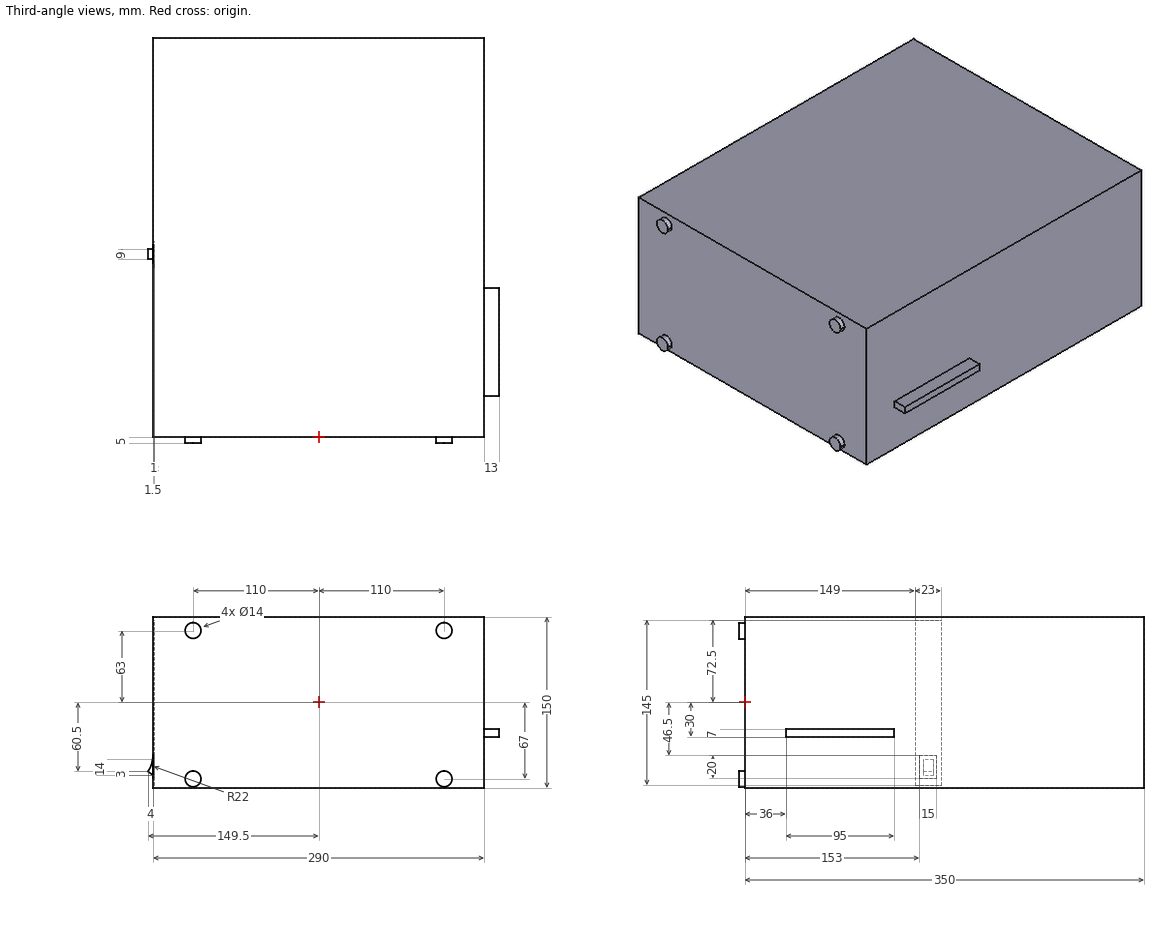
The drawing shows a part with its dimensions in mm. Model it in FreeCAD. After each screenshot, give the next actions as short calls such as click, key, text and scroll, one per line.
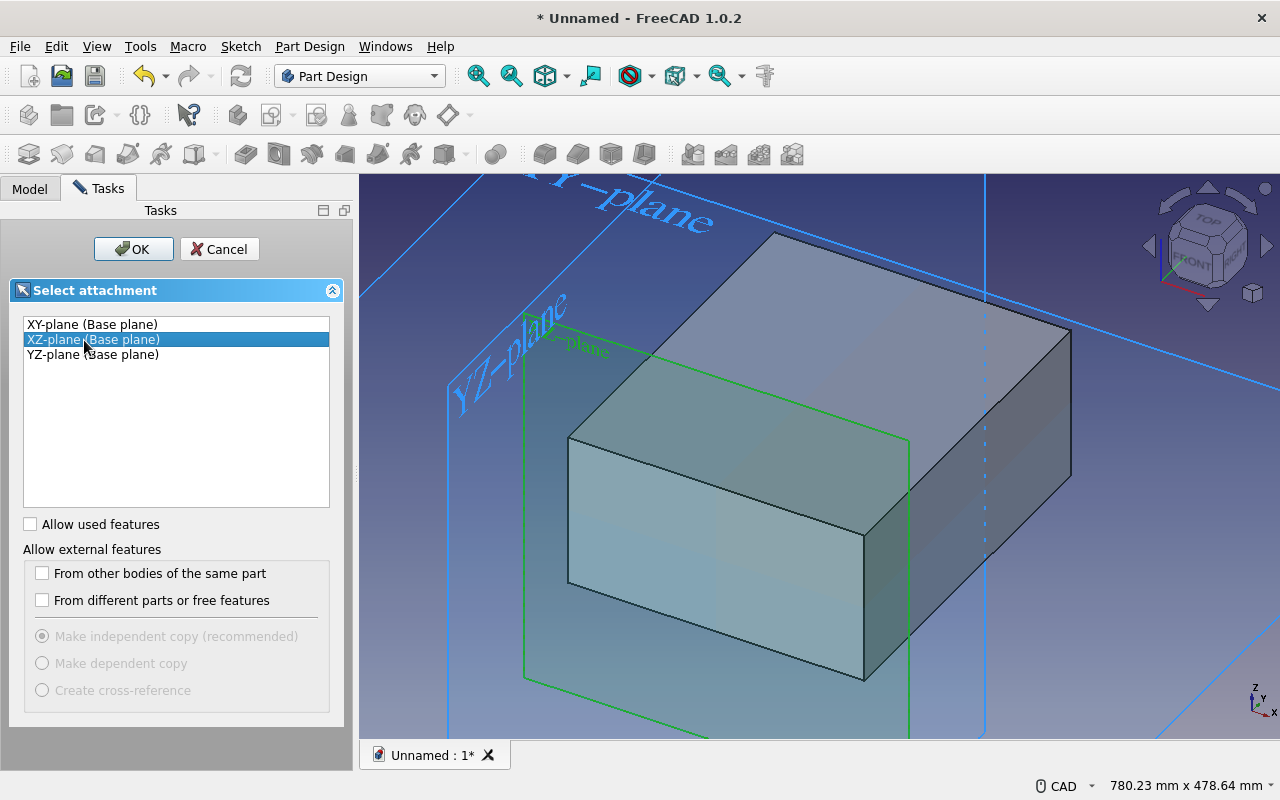
click(134, 249)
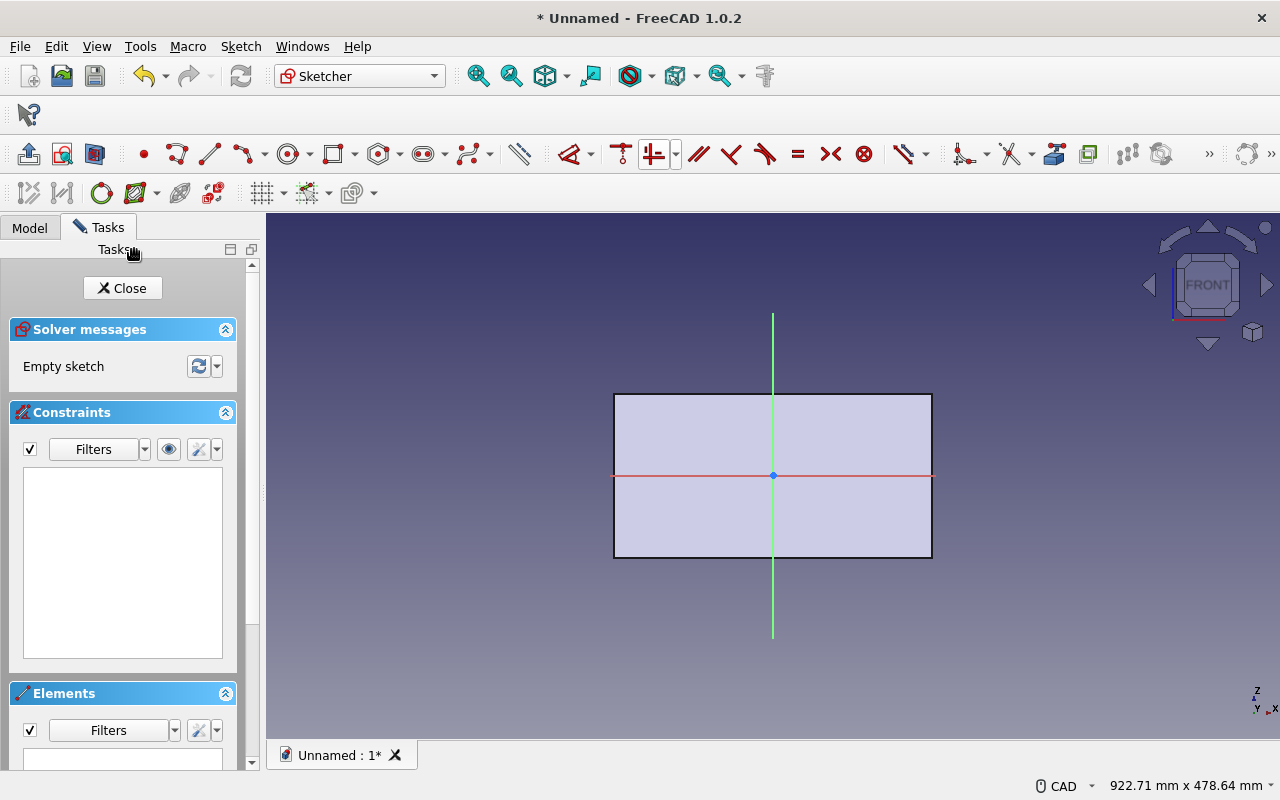
scroll(829, 480, up, 4)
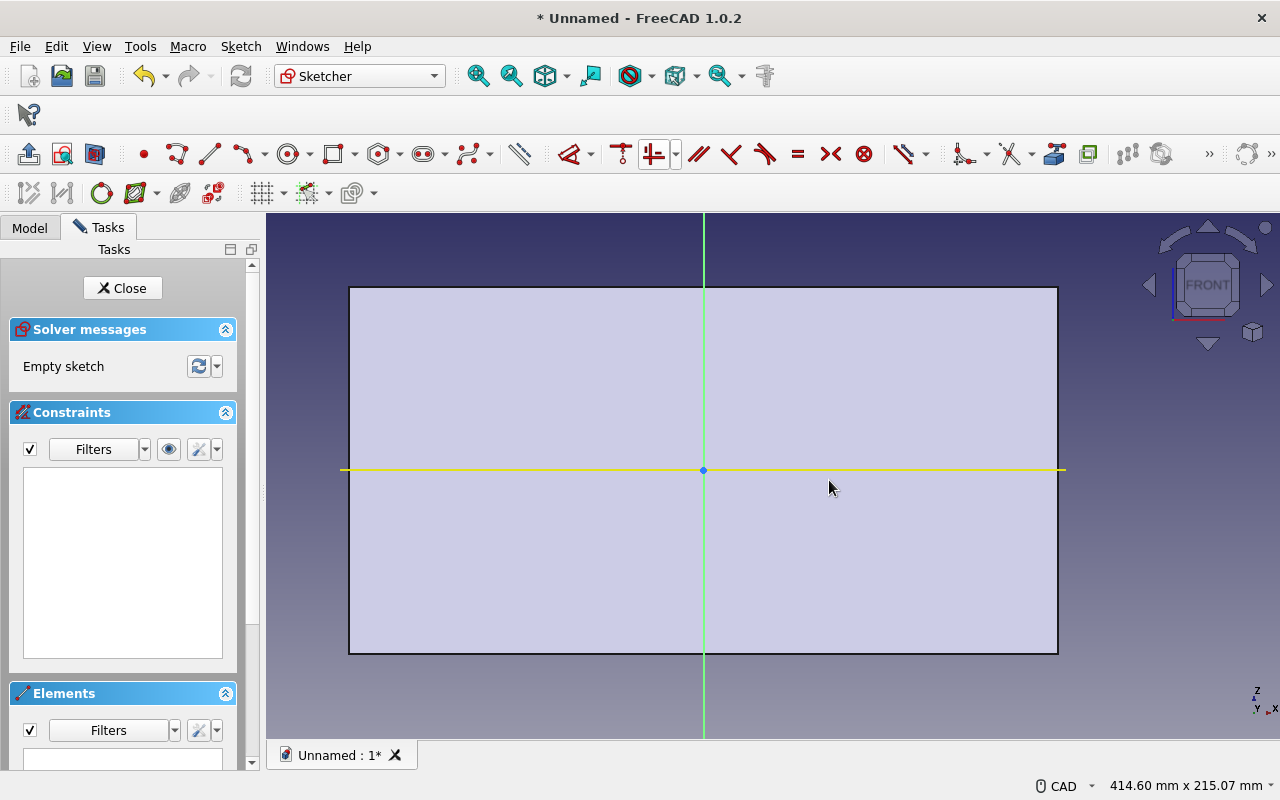
click(288, 154)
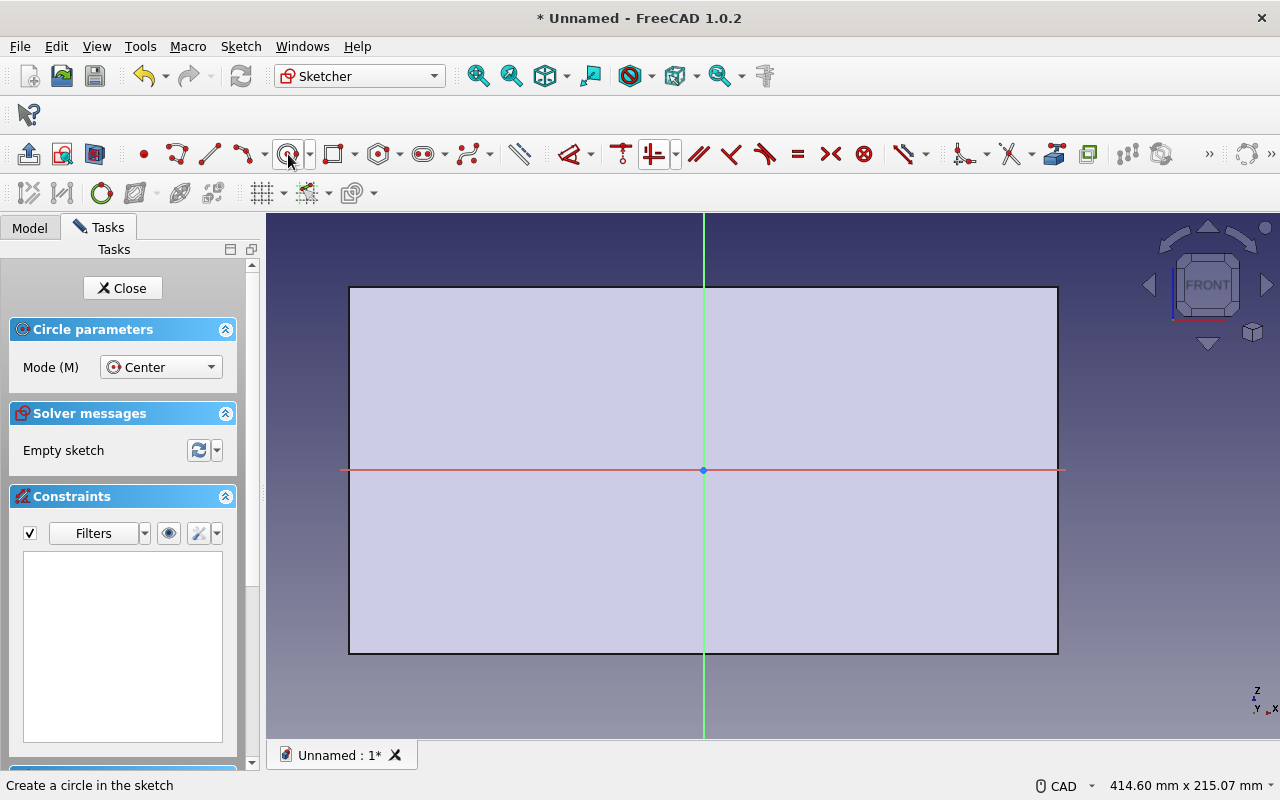
scroll(435, 316, up, 2)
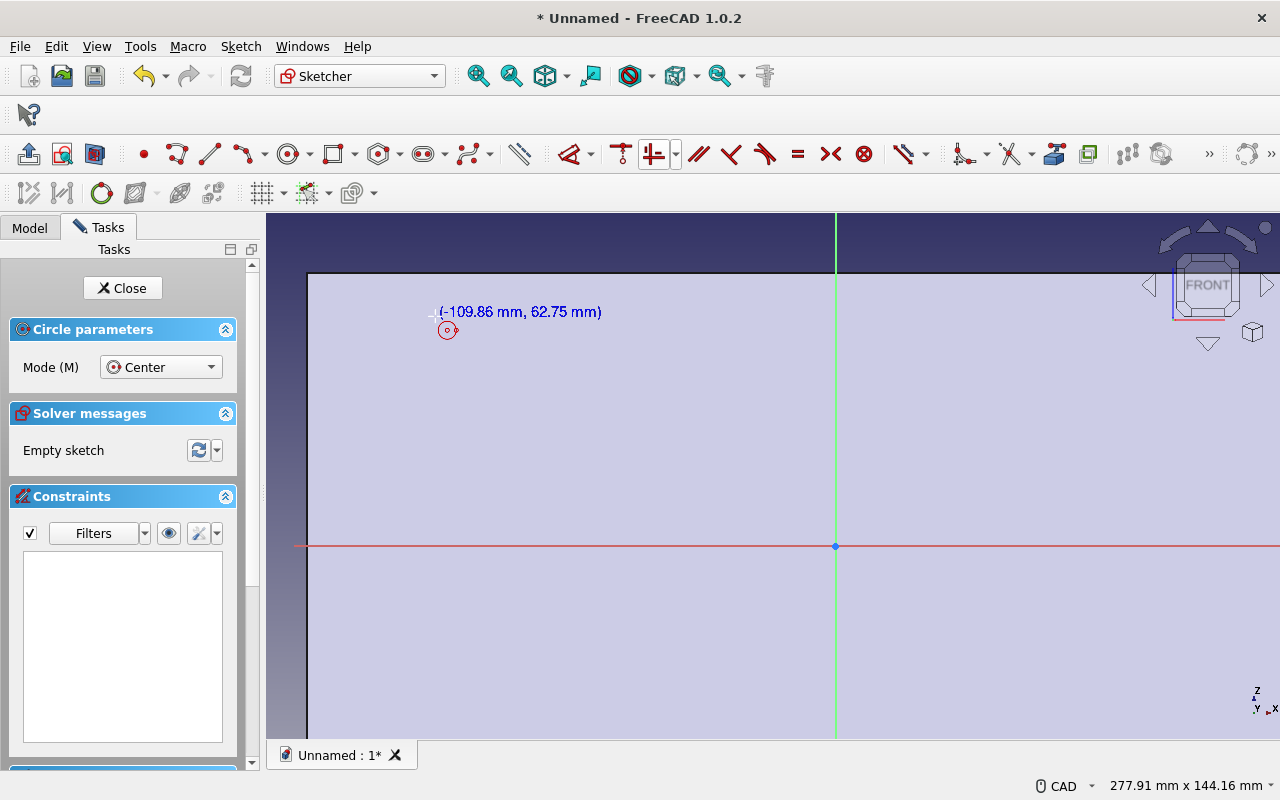
click(434, 316)
click(452, 298)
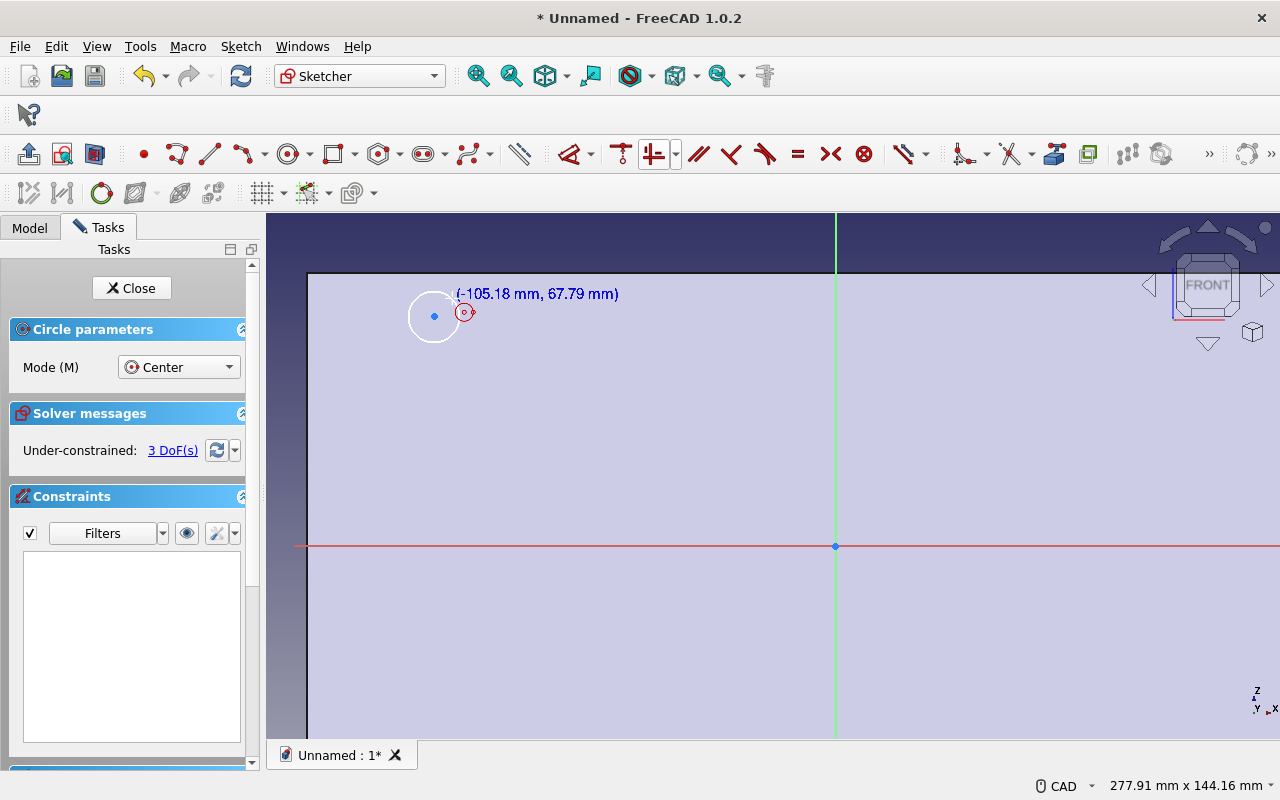
scroll(438, 318, down, 2)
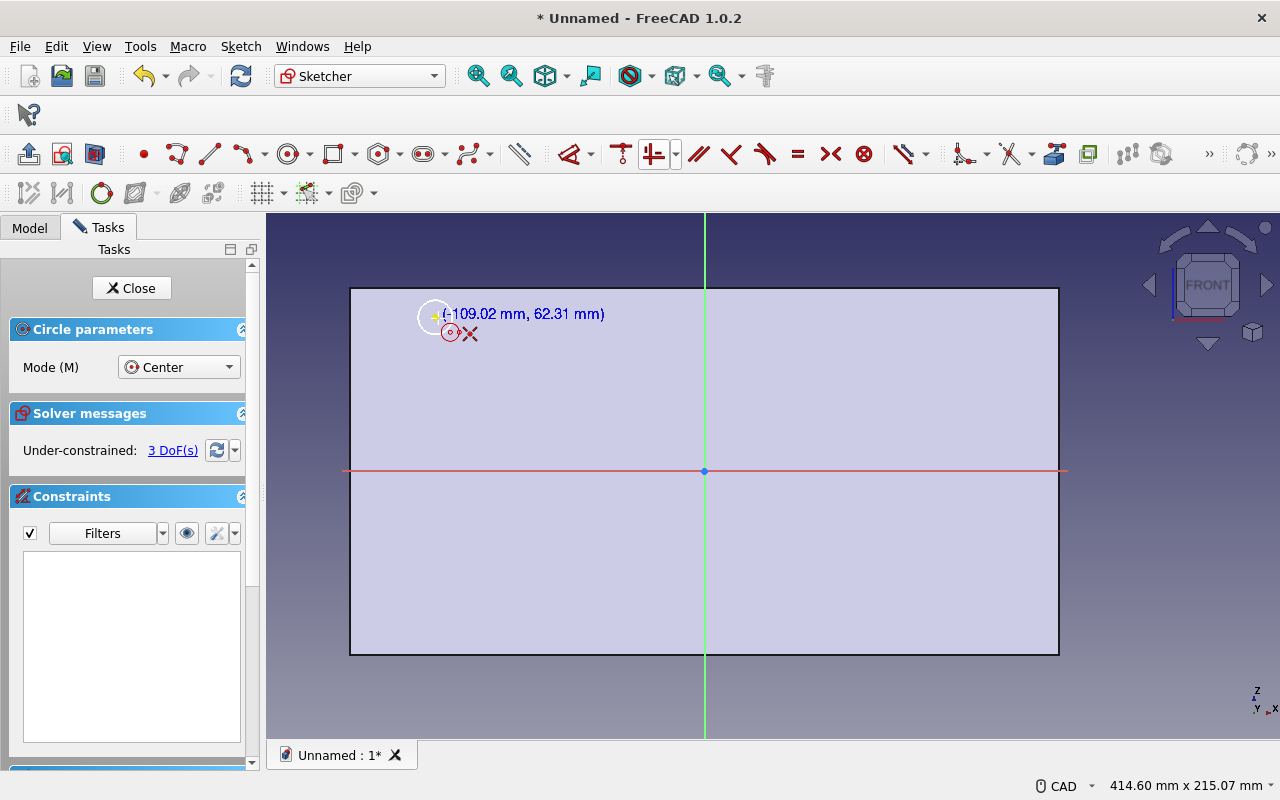
scroll(974, 317, up, 2)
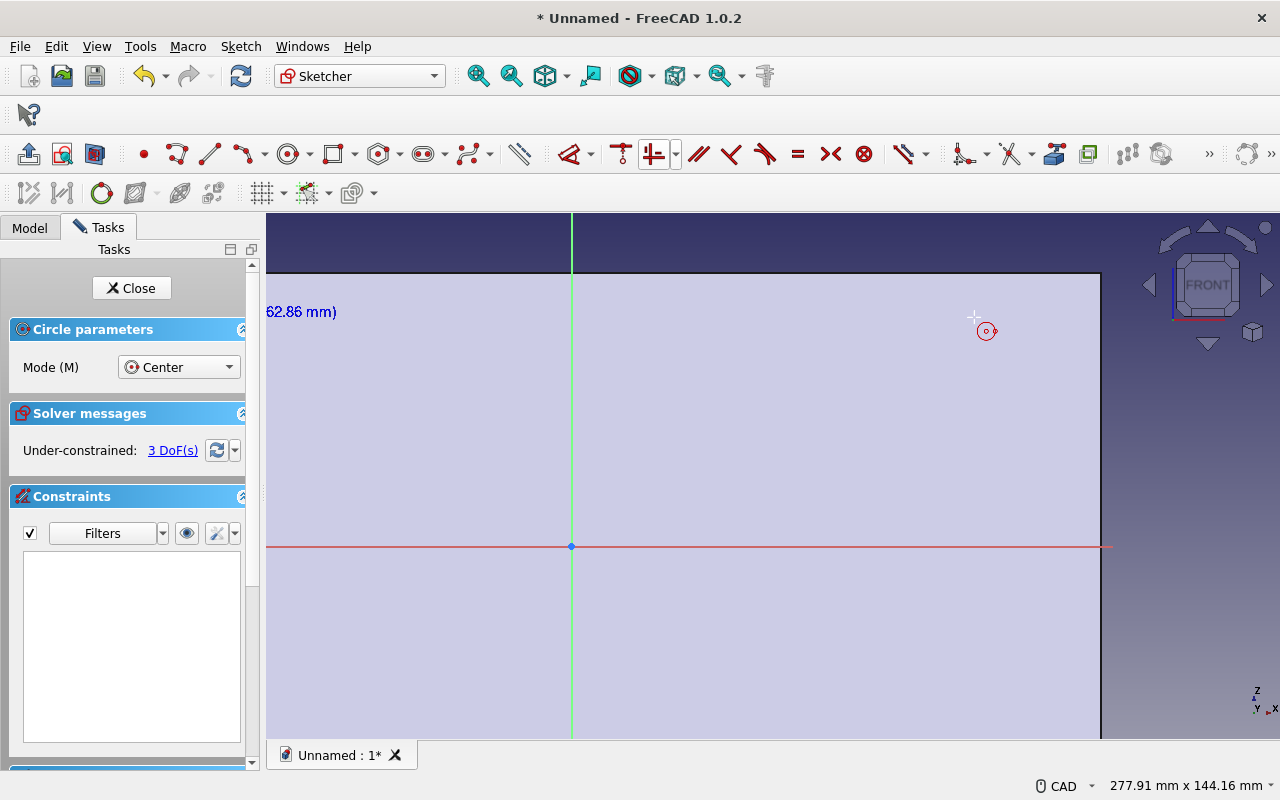
click(973, 317)
click(991, 299)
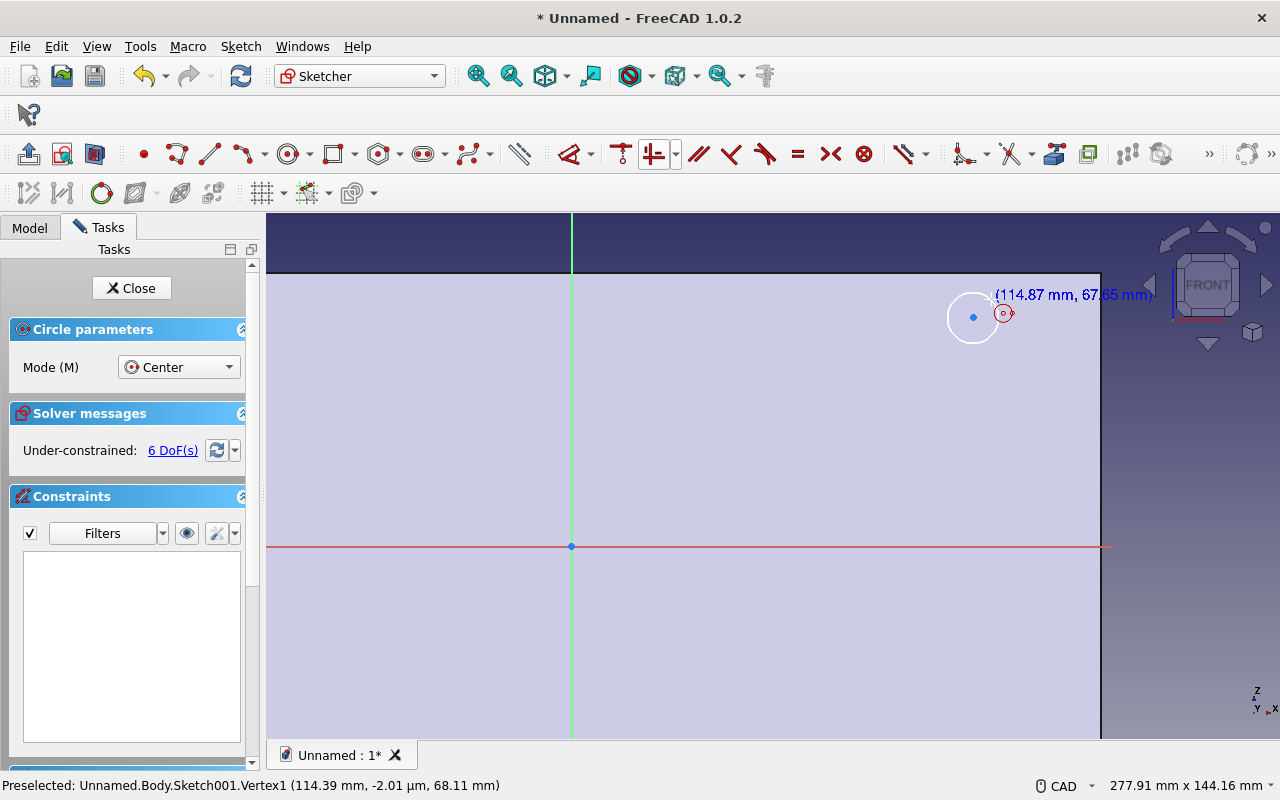
scroll(974, 317, down, 2)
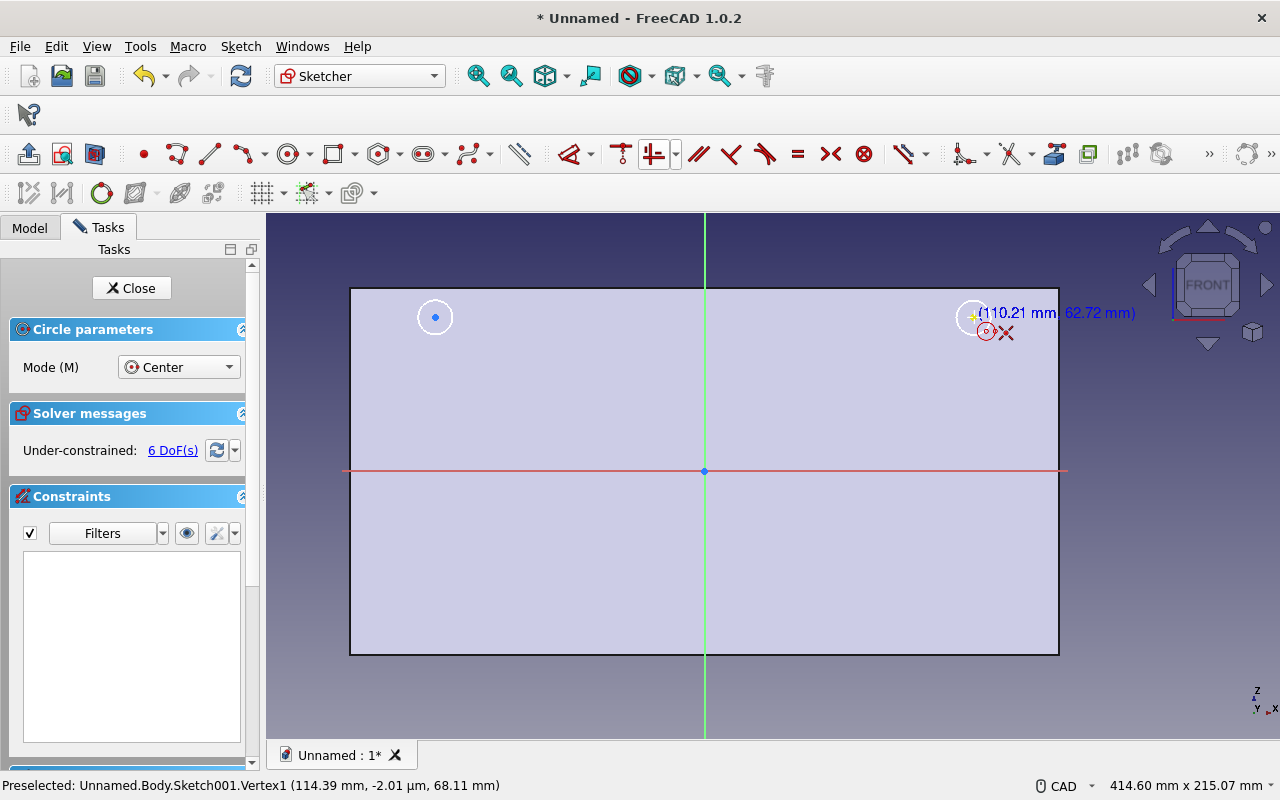
scroll(974, 635, up, 2)